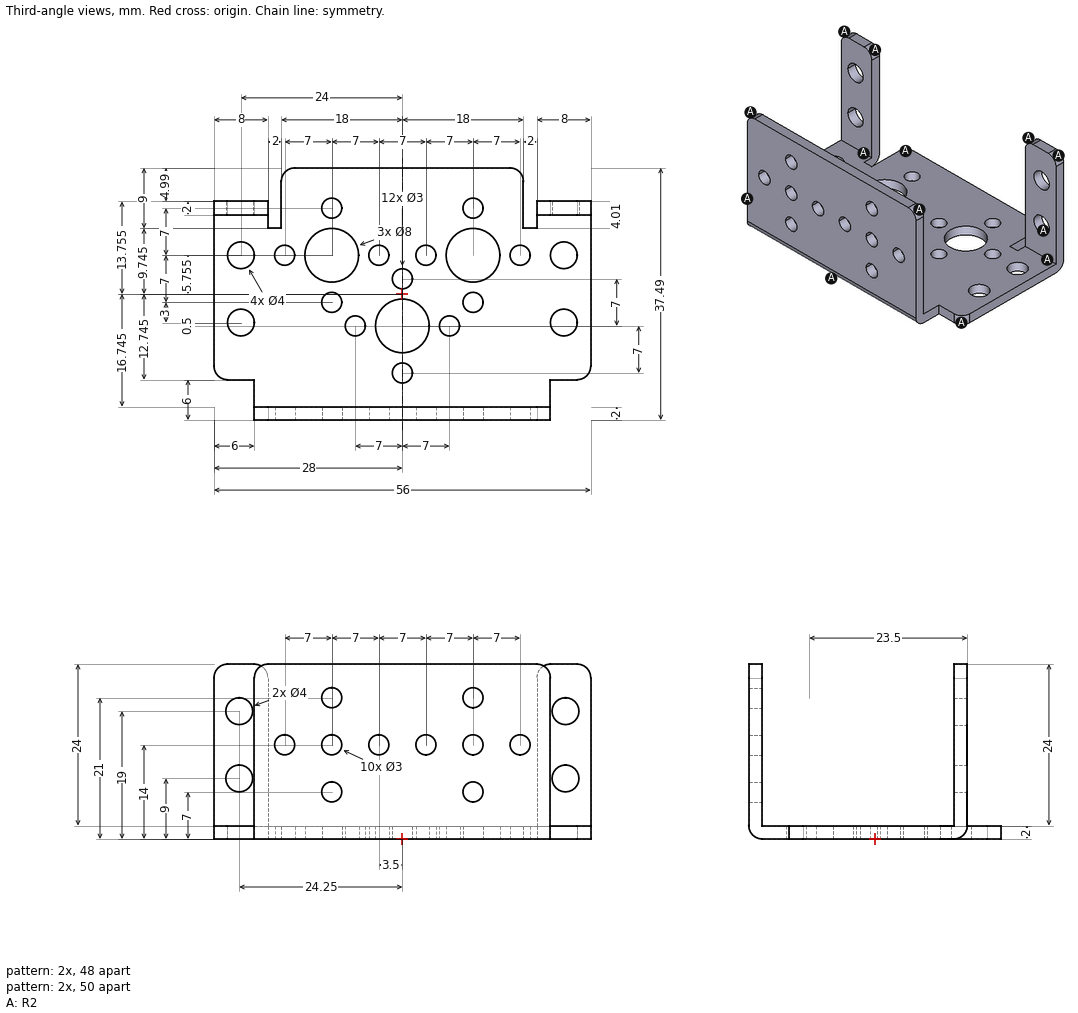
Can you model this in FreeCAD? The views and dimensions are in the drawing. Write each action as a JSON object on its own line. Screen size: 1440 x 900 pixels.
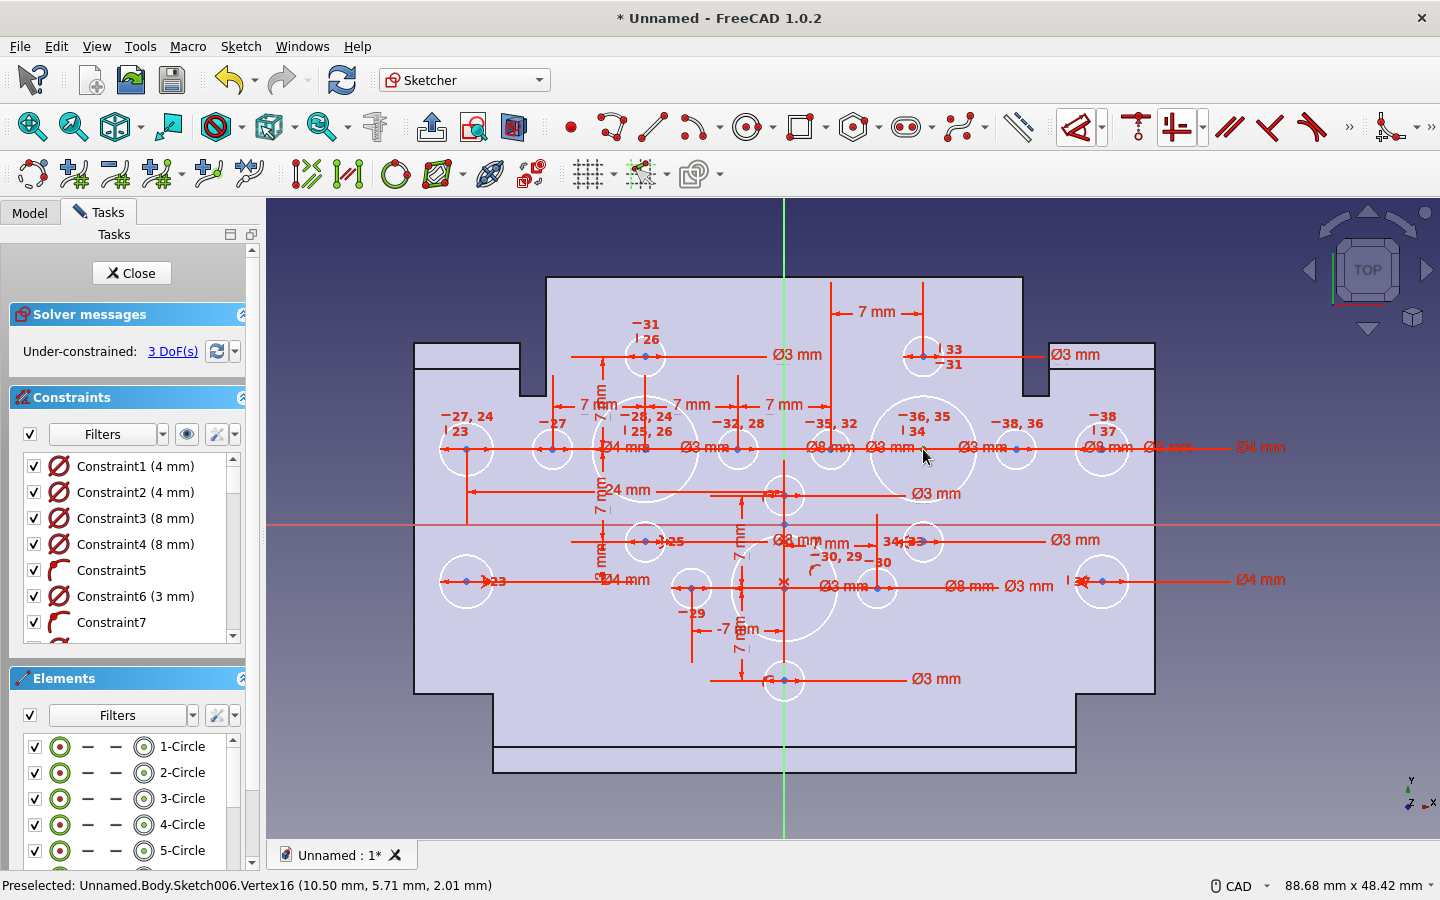
{"action": "left_click", "coordinate": [1016, 449]}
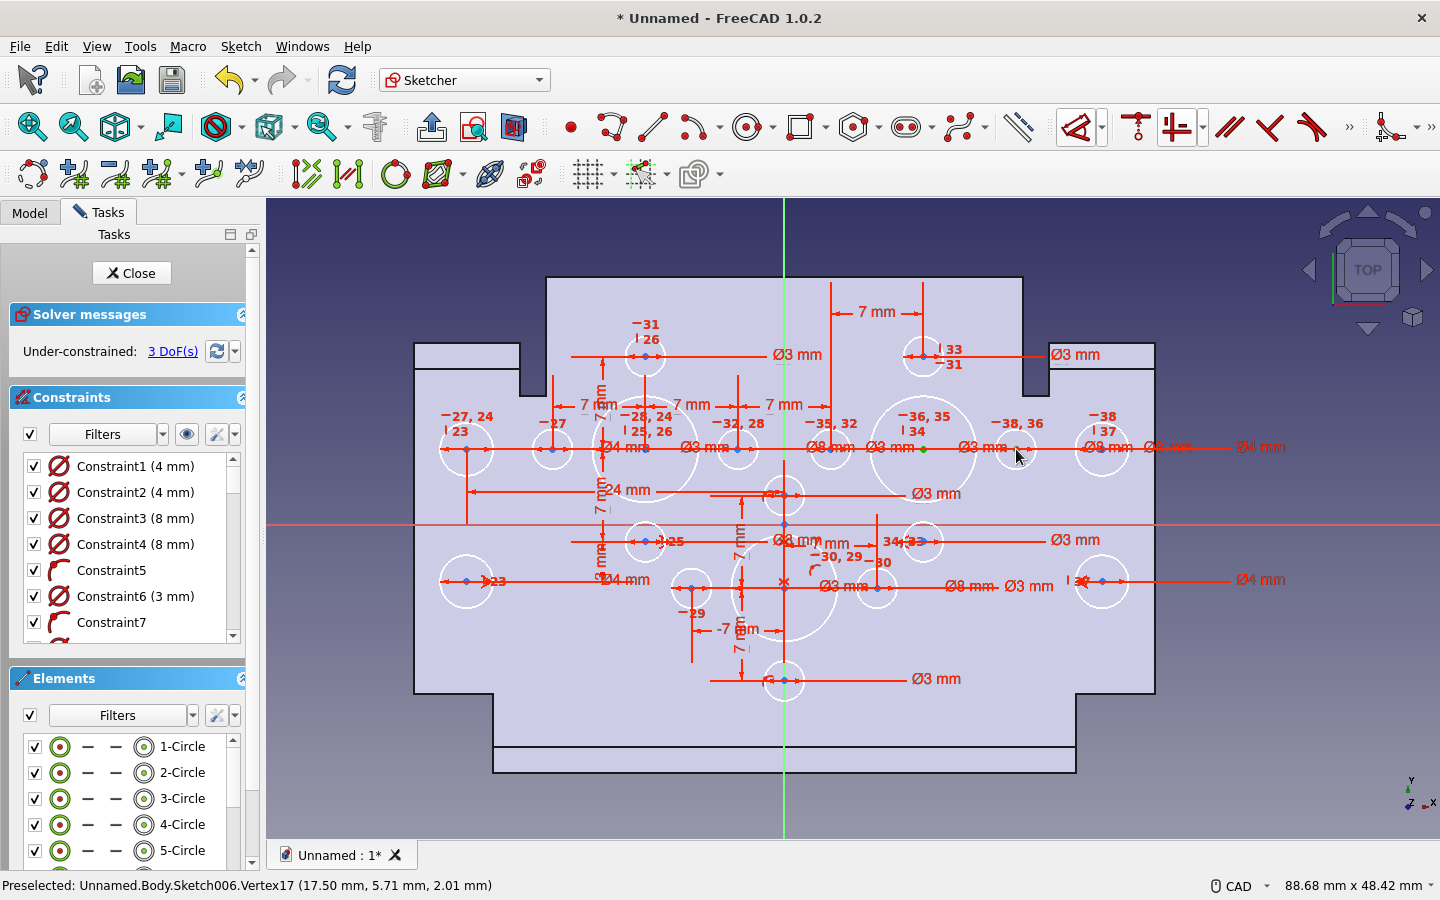
{"action": "key", "text": "l"}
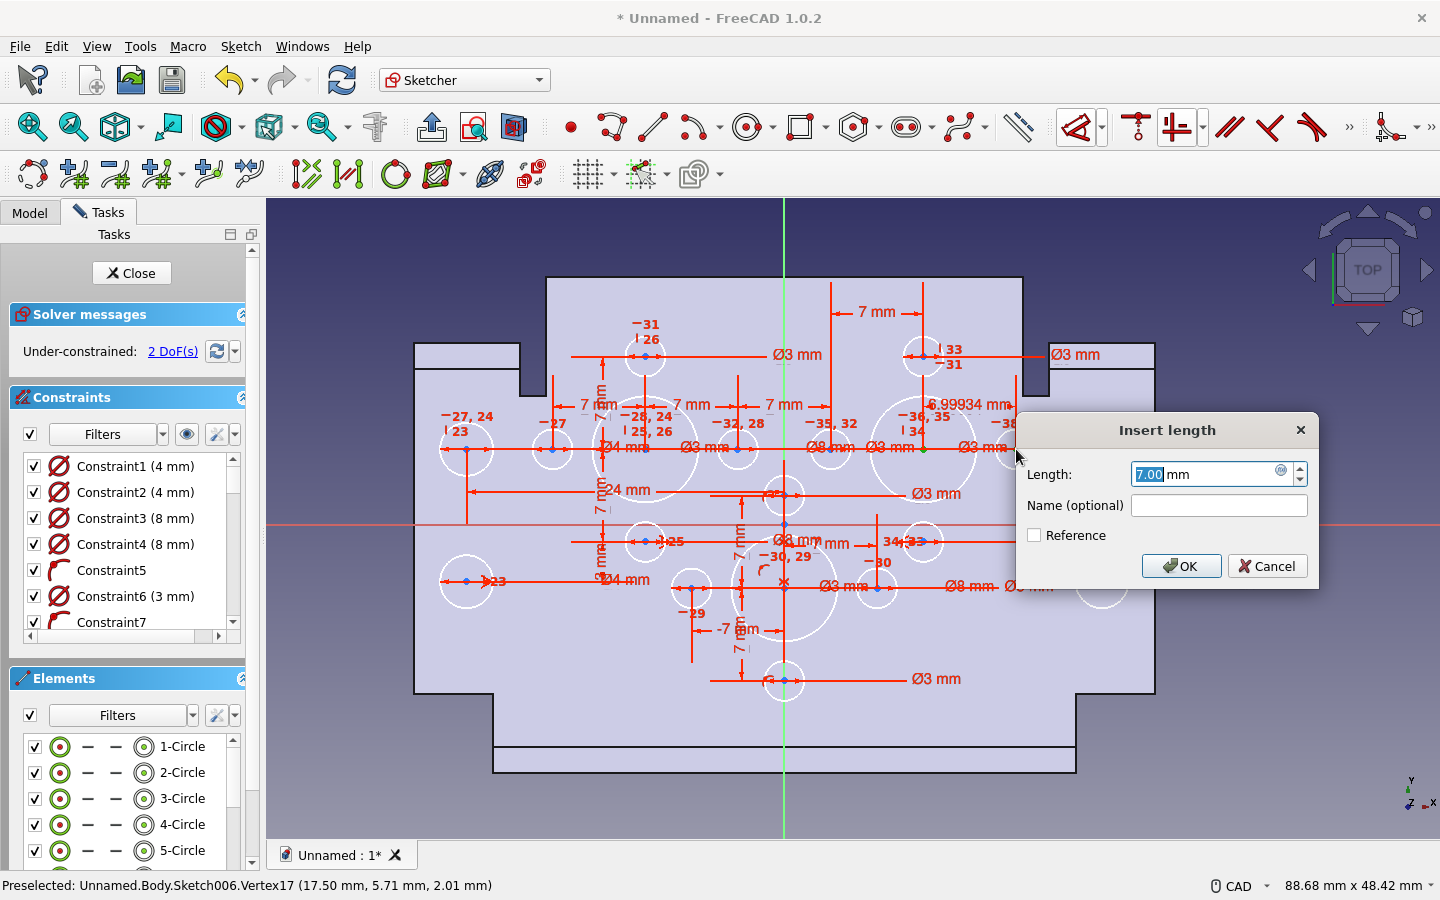
{"action": "type", "text": "7"}
{"action": "key", "text": "Return"}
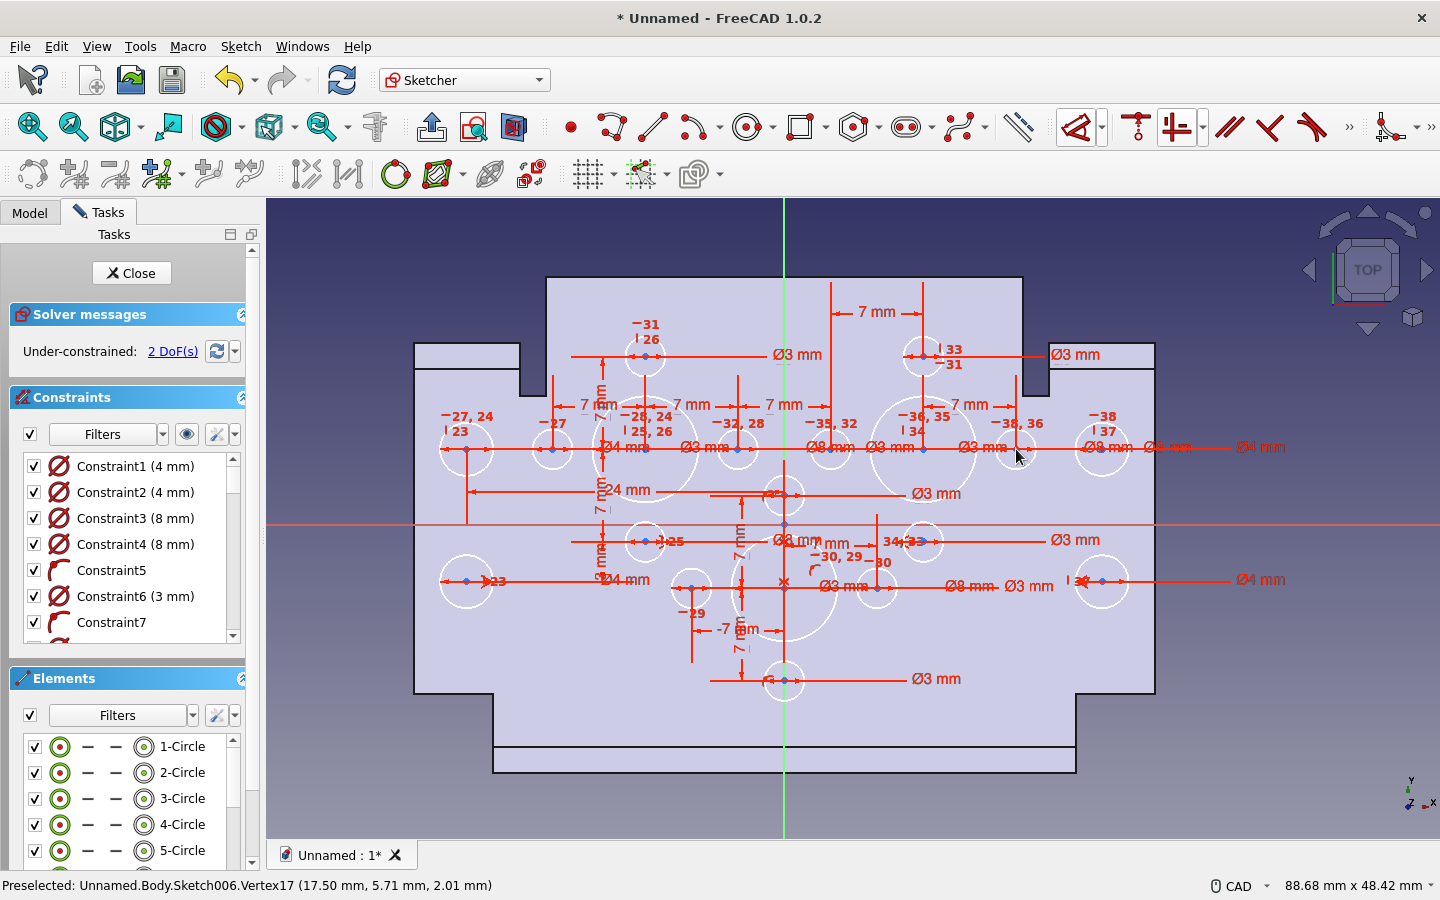
{"action": "scroll", "coordinate": [467, 582], "scroll_direction": "up", "scroll_amount": 9}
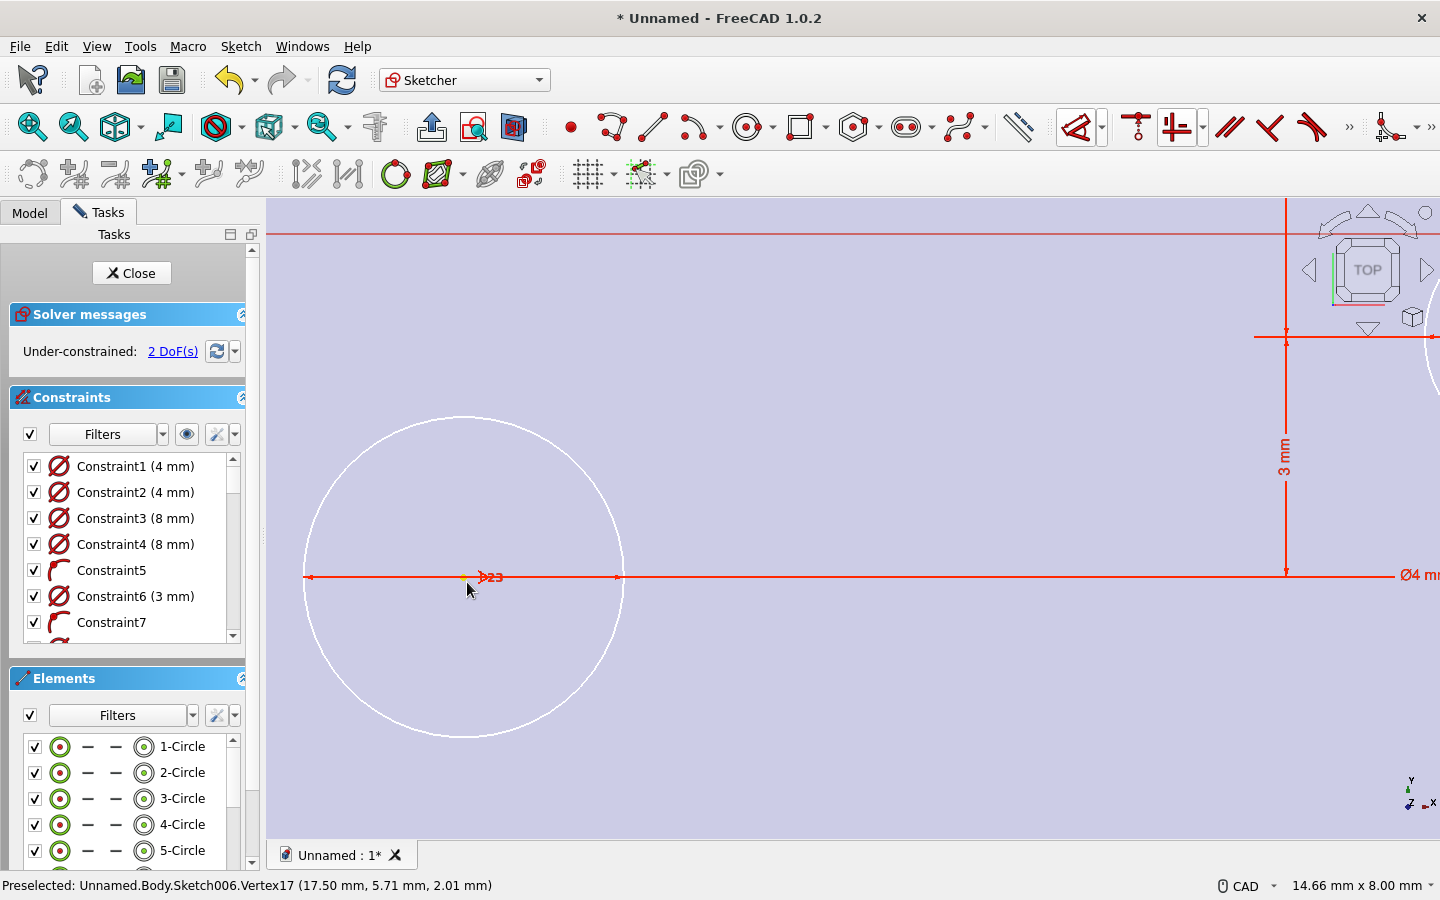
{"action": "left_click", "coordinate": [464, 577]}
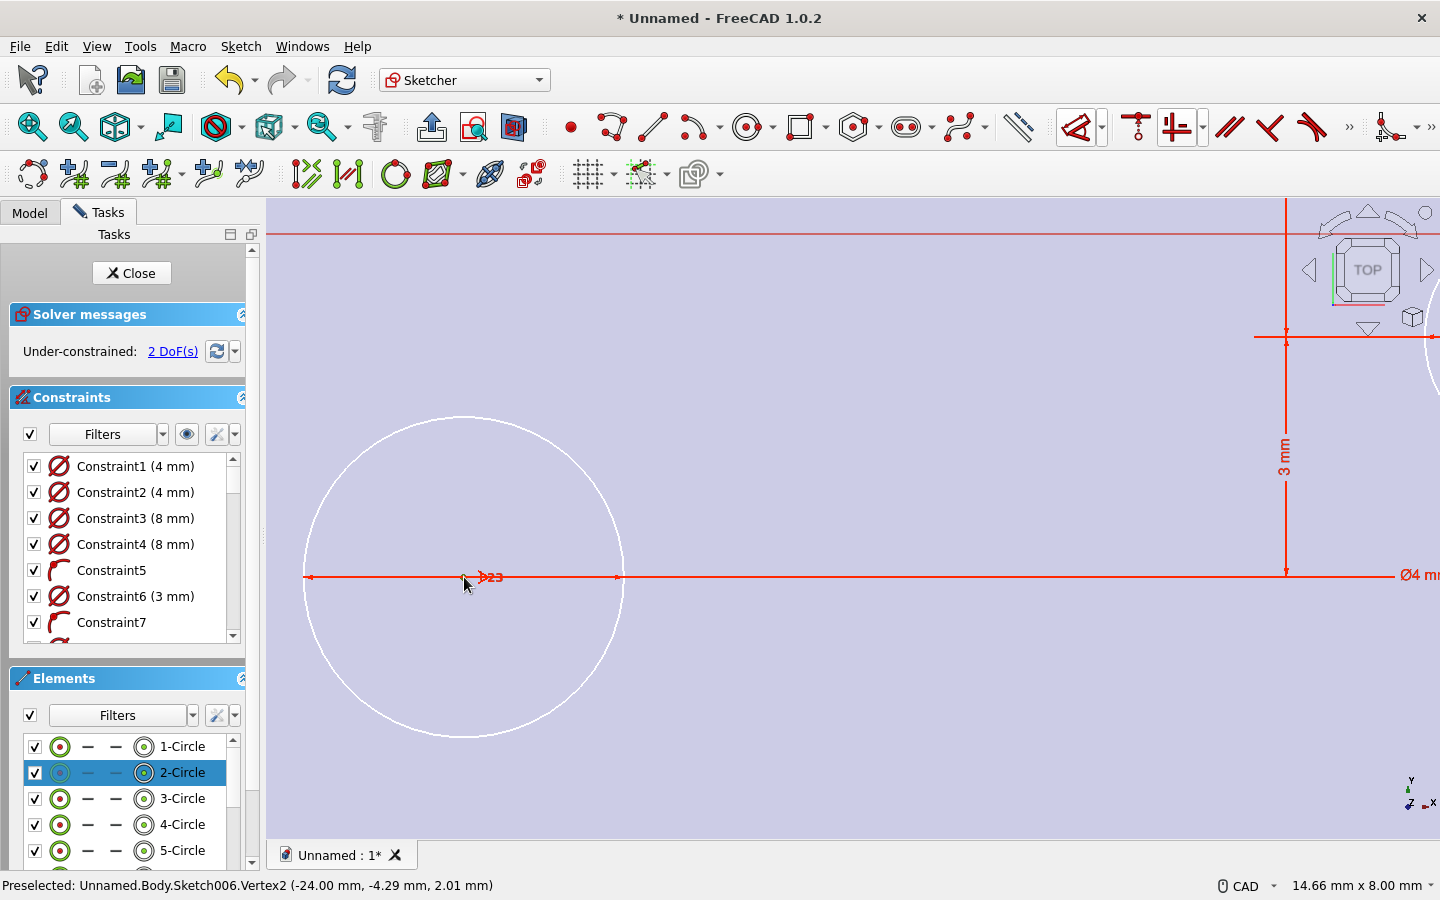
{"action": "scroll", "coordinate": [467, 583], "scroll_direction": "down", "scroll_amount": 9}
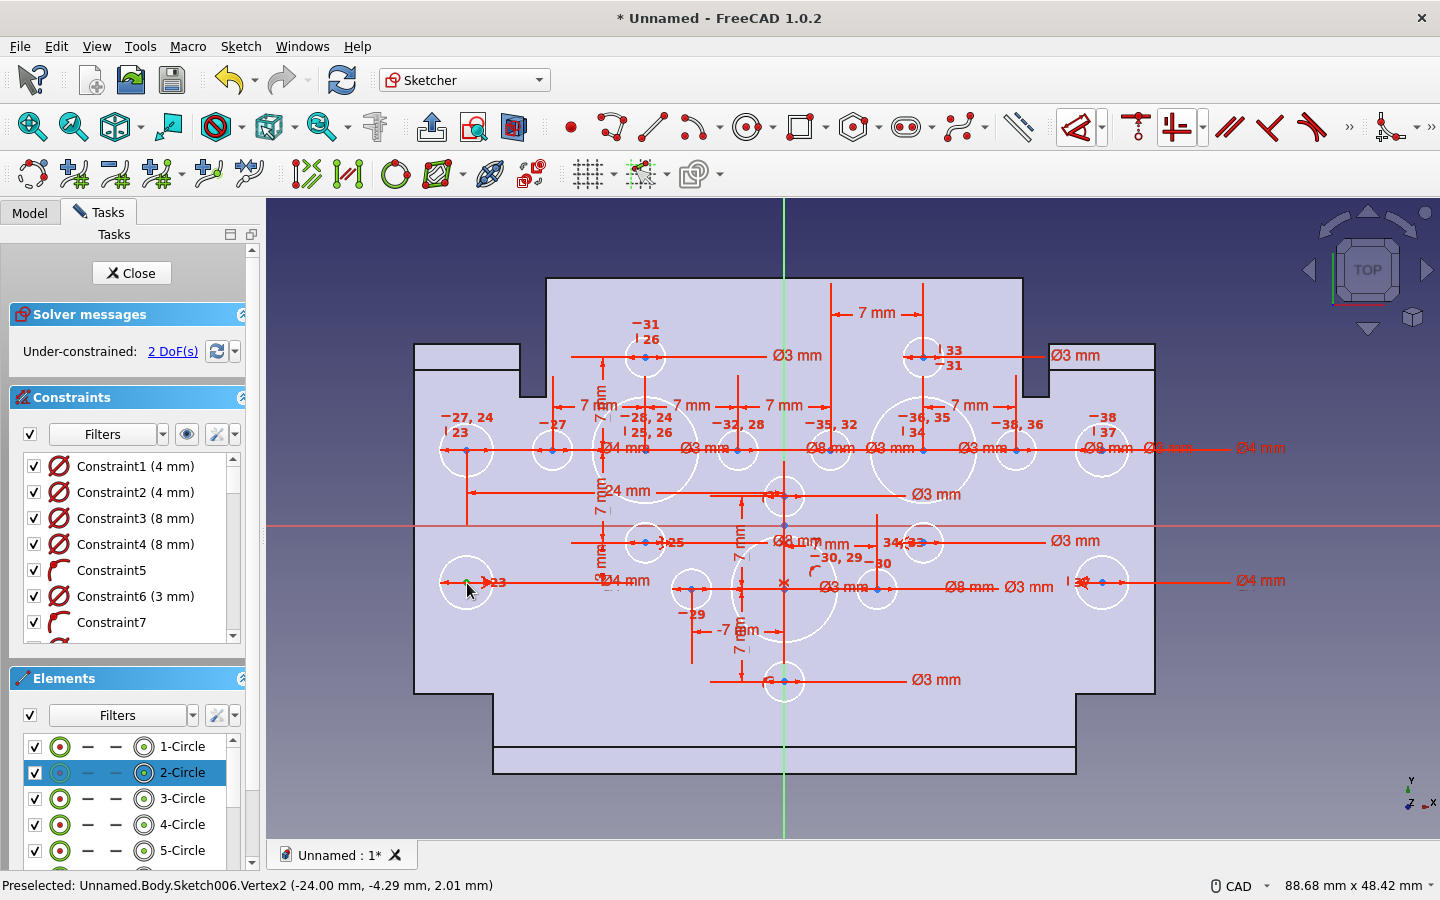
{"action": "scroll", "coordinate": [784, 589], "scroll_direction": "up", "scroll_amount": 9}